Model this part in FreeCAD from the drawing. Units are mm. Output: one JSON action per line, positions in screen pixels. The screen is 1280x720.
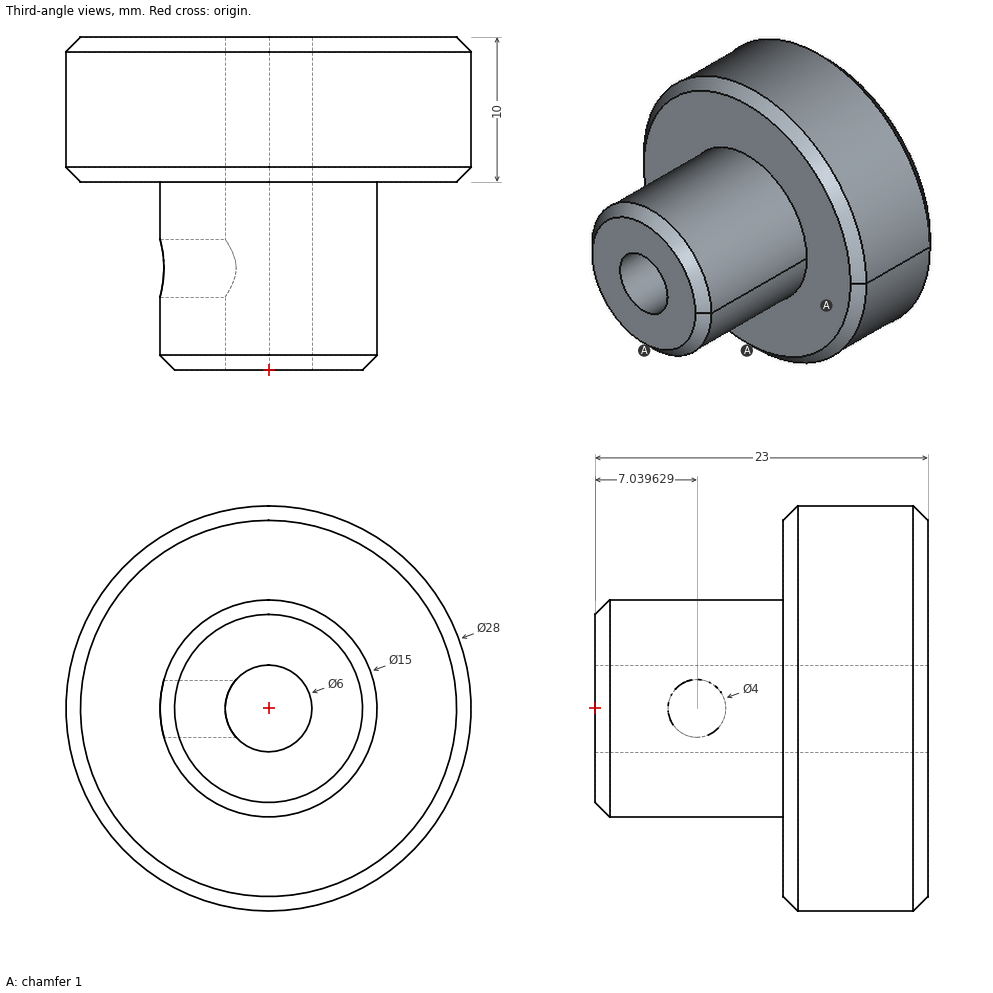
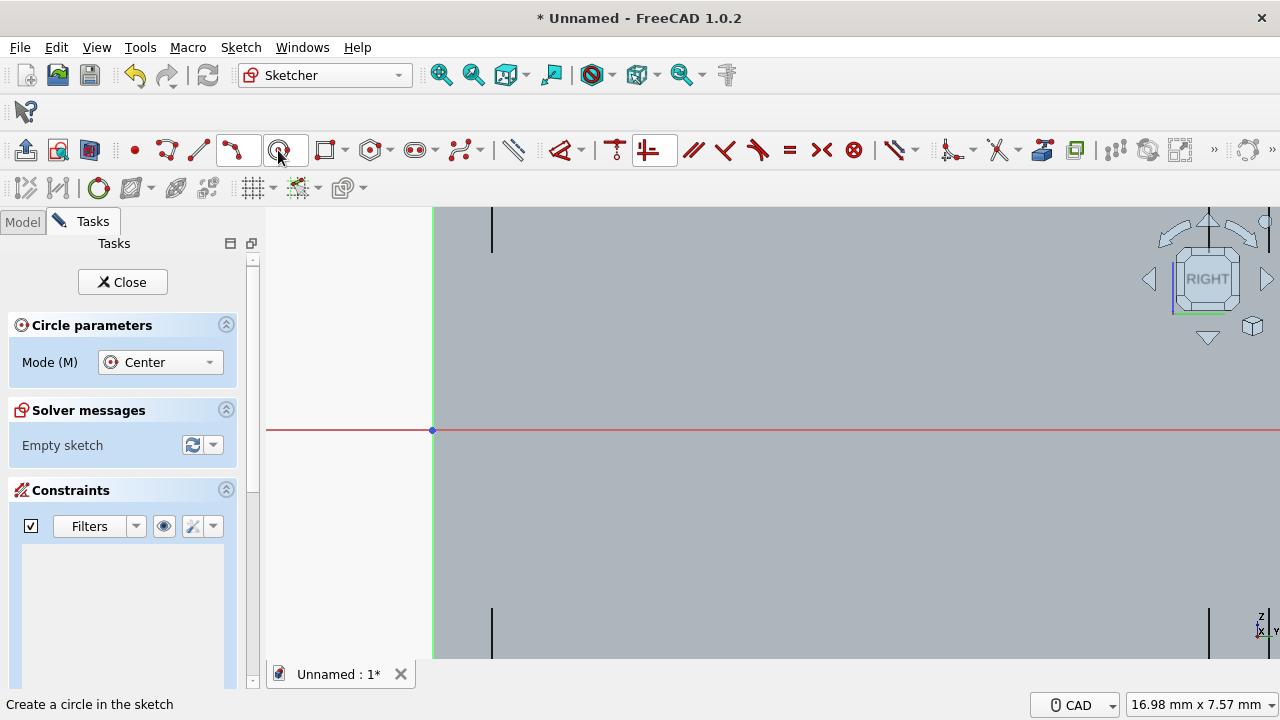
{"action": "left_click", "coordinate": [853, 430]}
{"action": "mouse_move", "coordinate": [937, 346]}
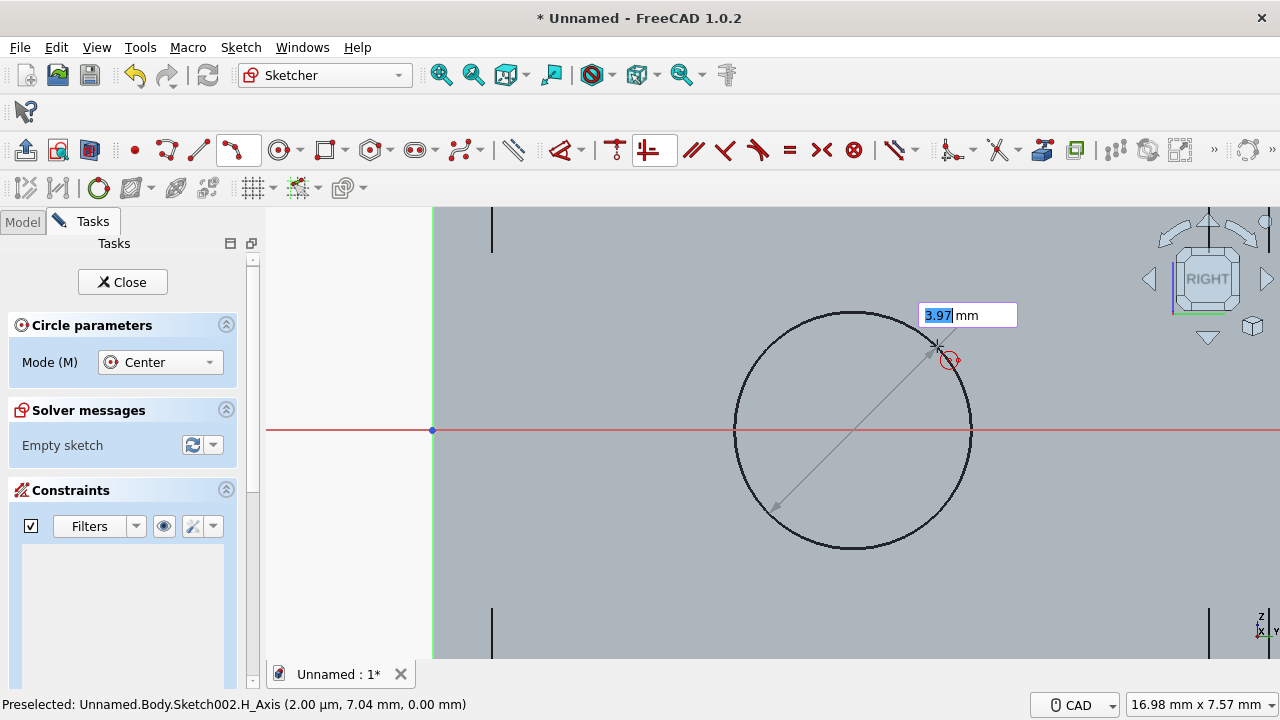
{"action": "type", "text": "4"}
{"action": "key", "text": "Return"}
{"action": "key", "text": "Escape"}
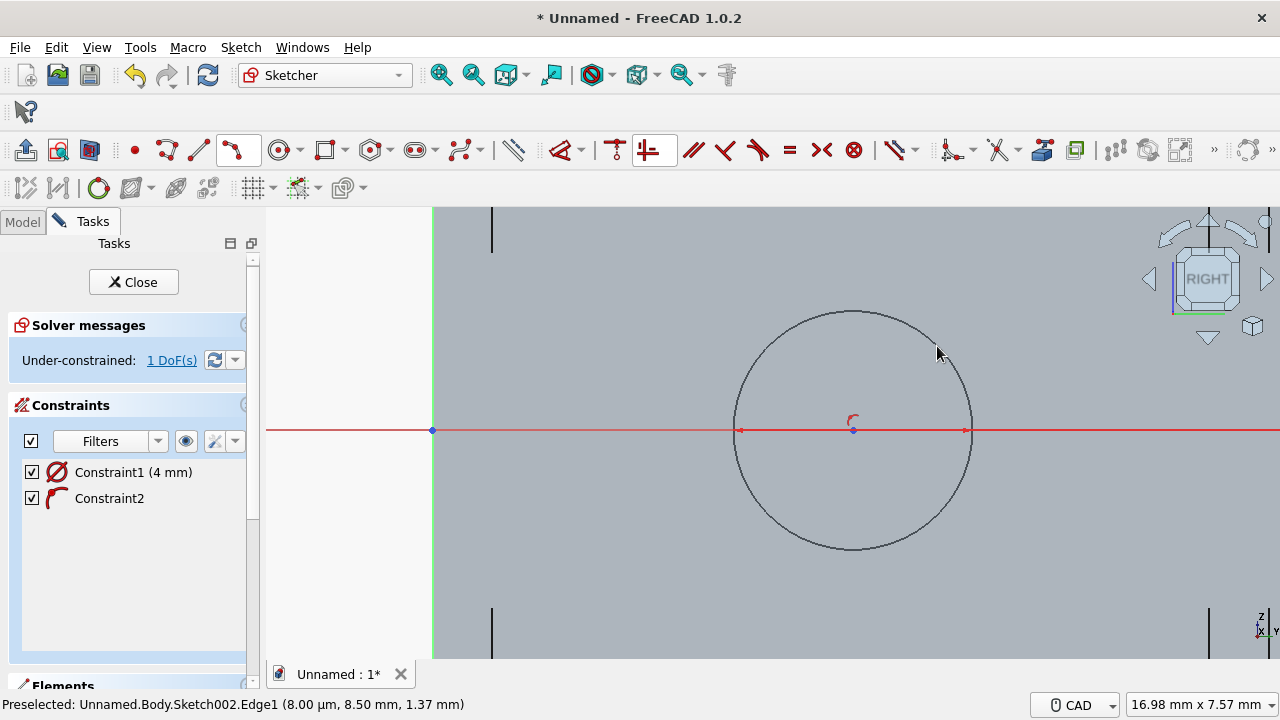
{"action": "key", "text": "d"}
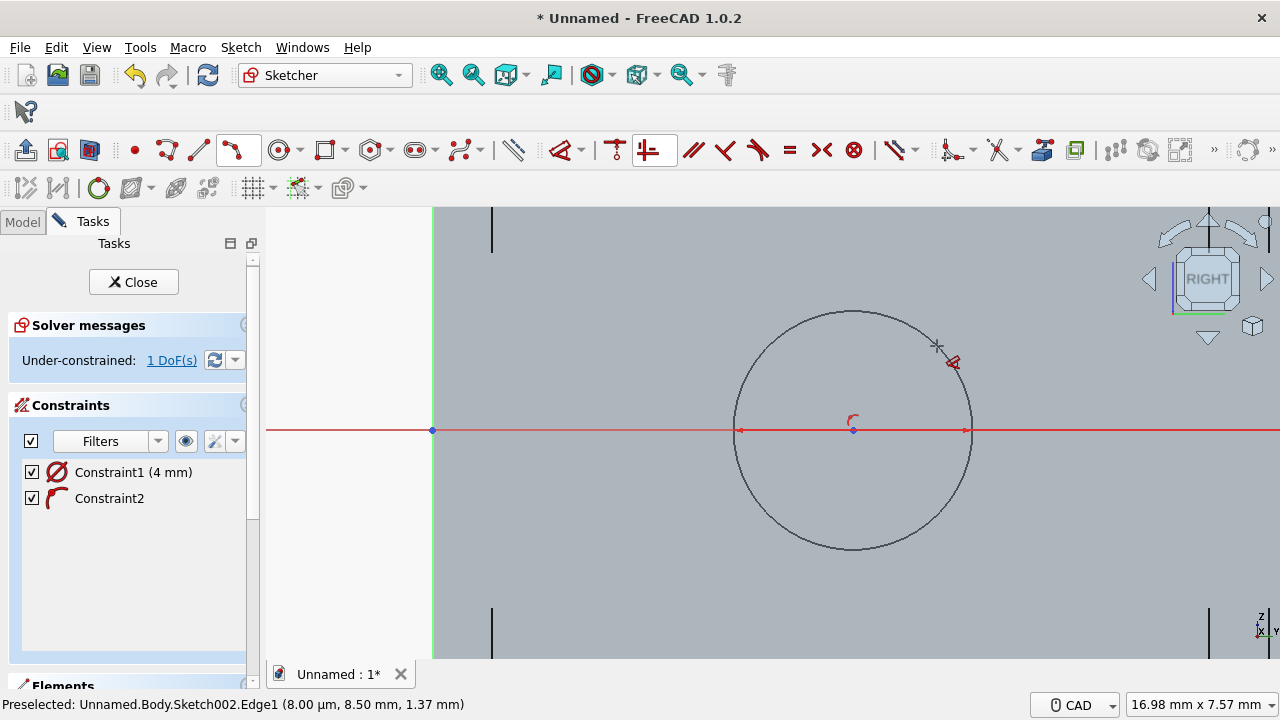
{"action": "left_click", "coordinate": [853, 430]}
{"action": "left_click", "coordinate": [643, 464]}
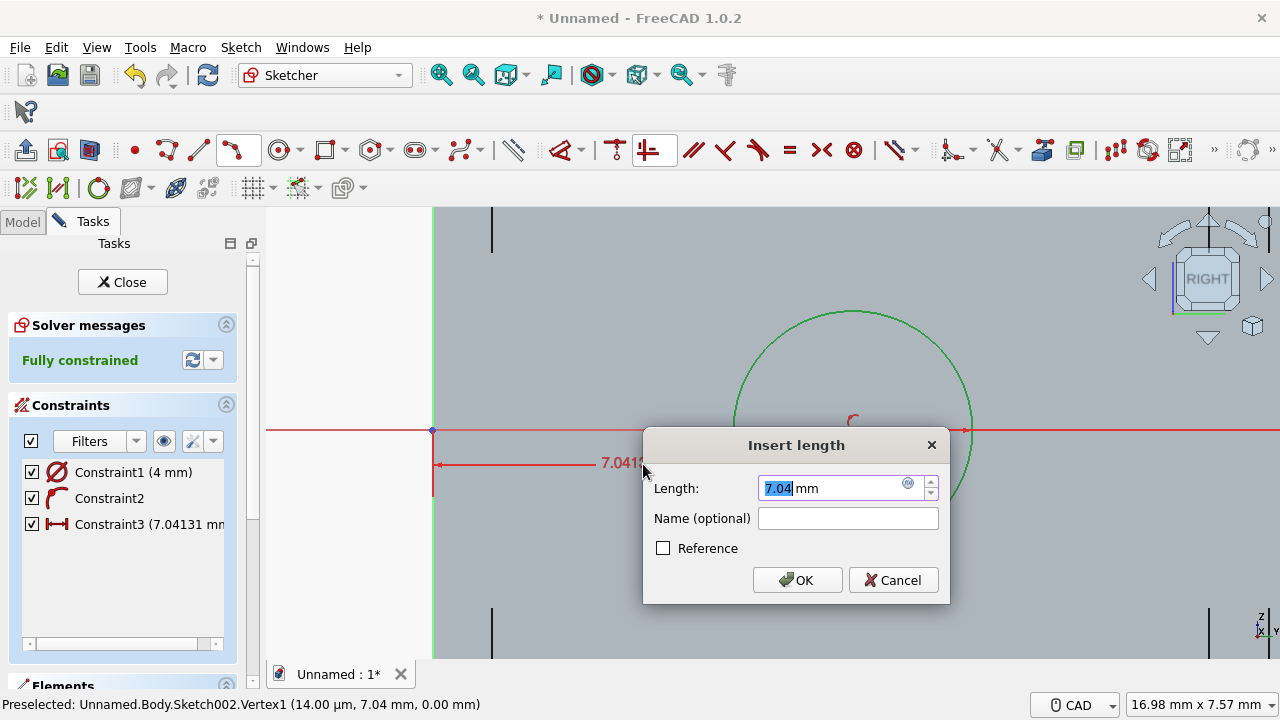
{"action": "type", "text": "7.039629"}
{"action": "key", "text": "Return"}
{"action": "key", "text": "Escape"}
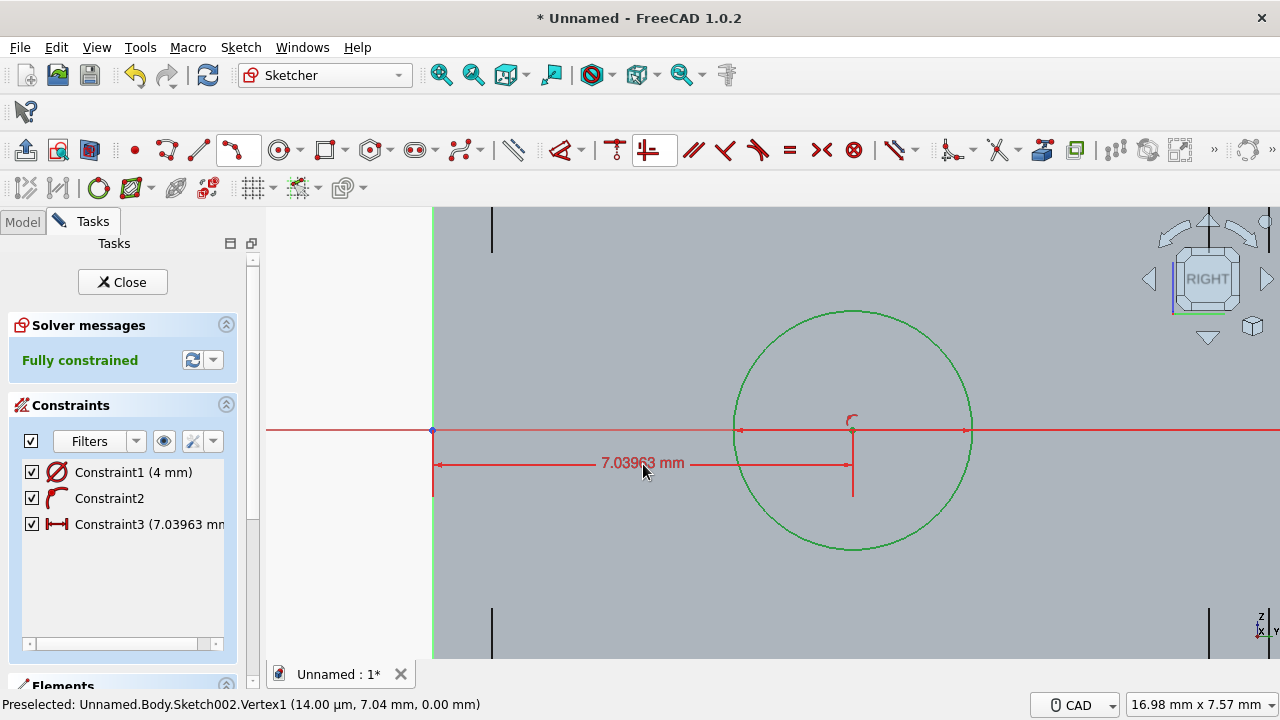
{"action": "left_click", "coordinate": [123, 282]}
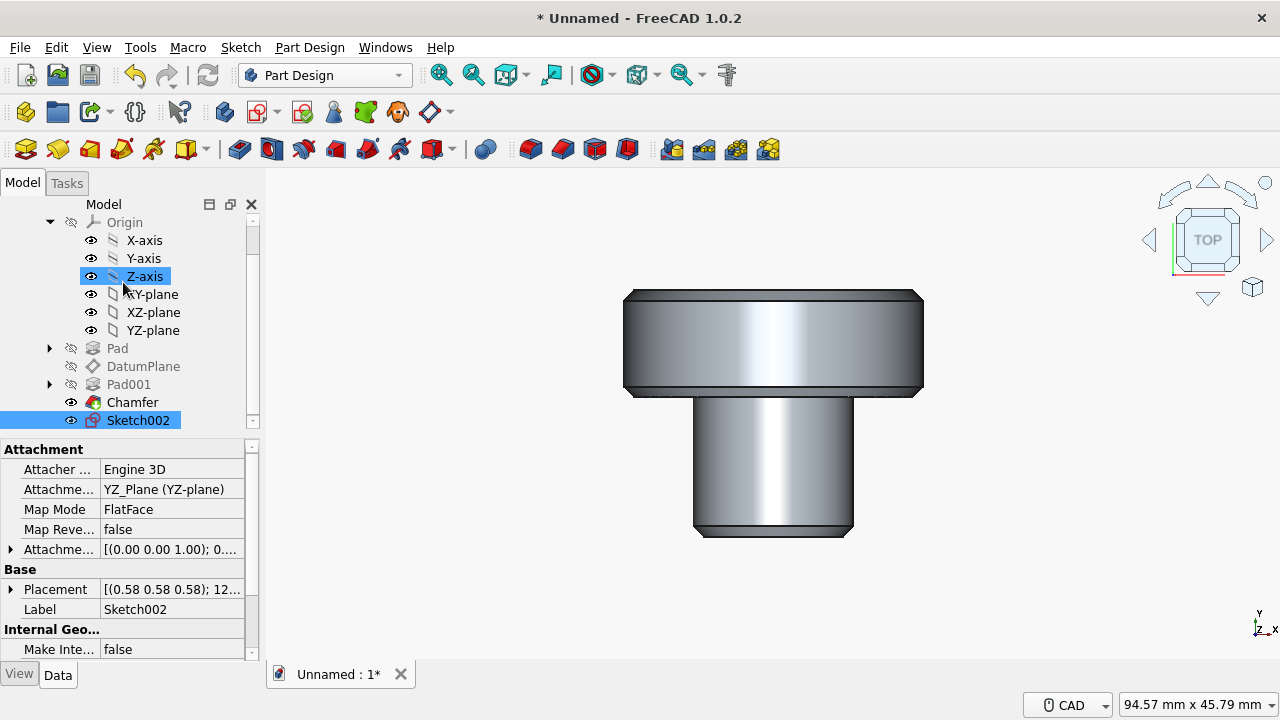
{"action": "left_click", "coordinate": [240, 150]}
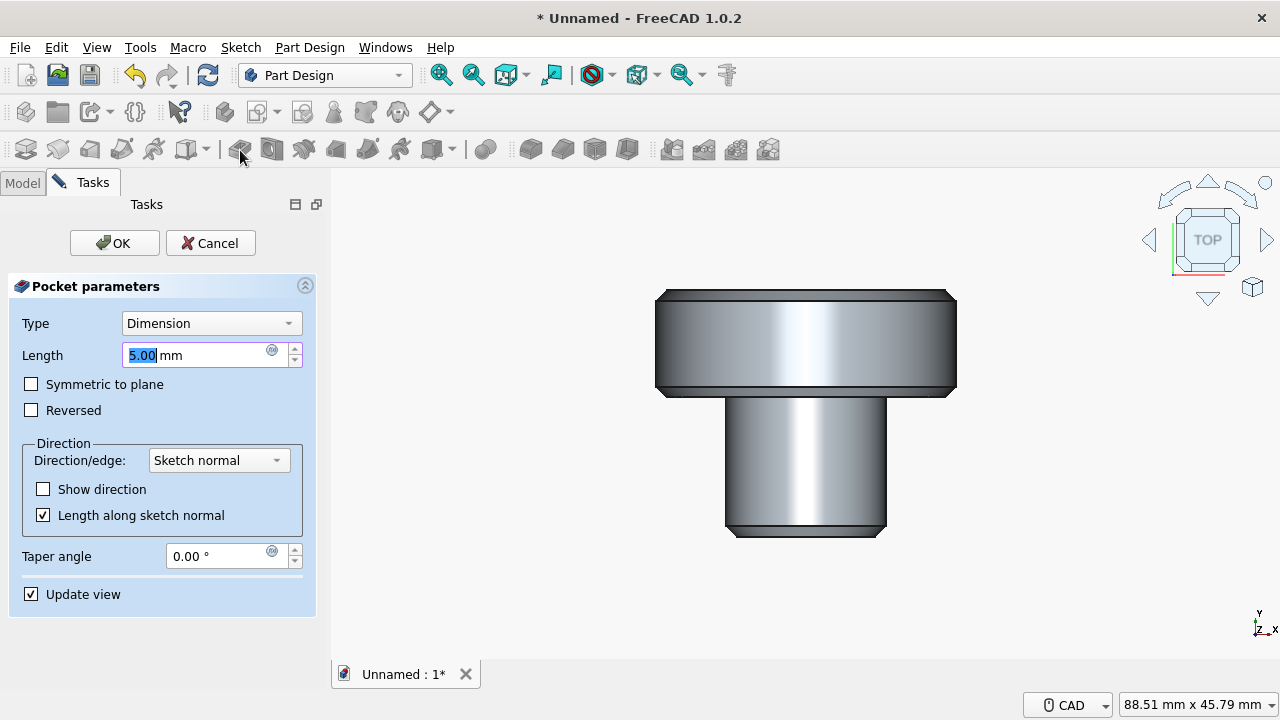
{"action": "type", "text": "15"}
{"action": "key", "text": "Tab"}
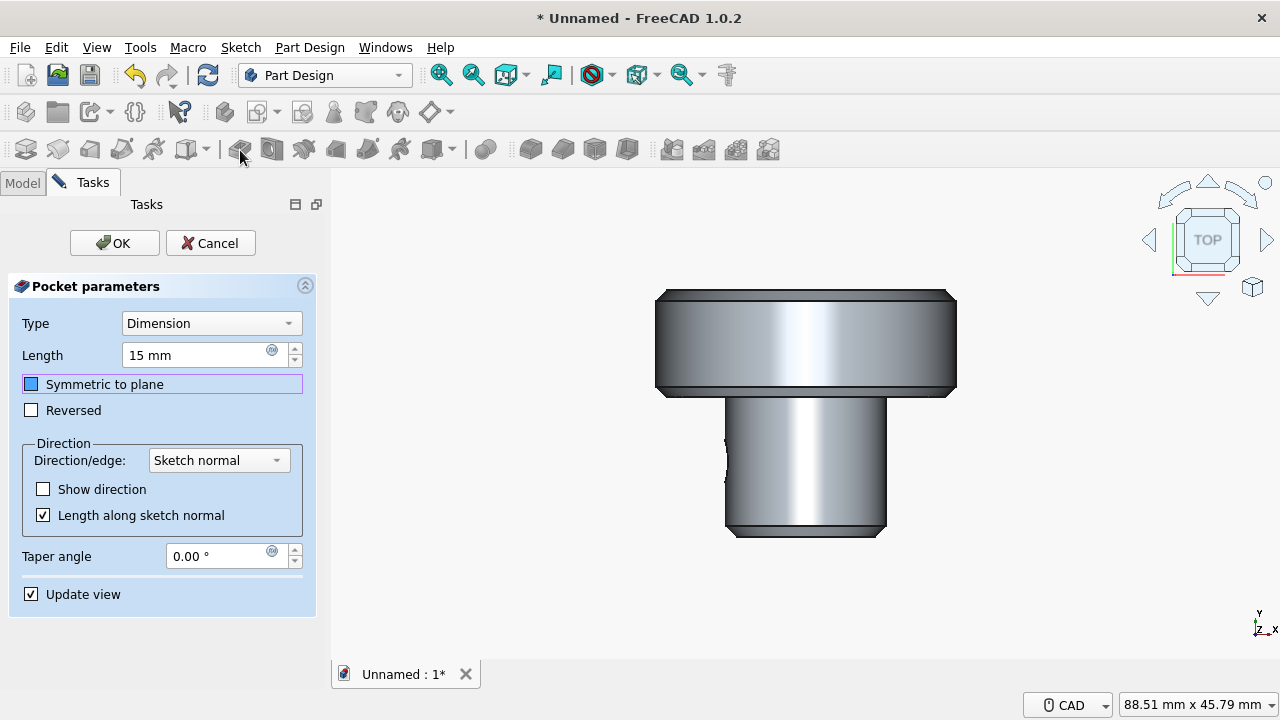
{"action": "left_click", "coordinate": [115, 243]}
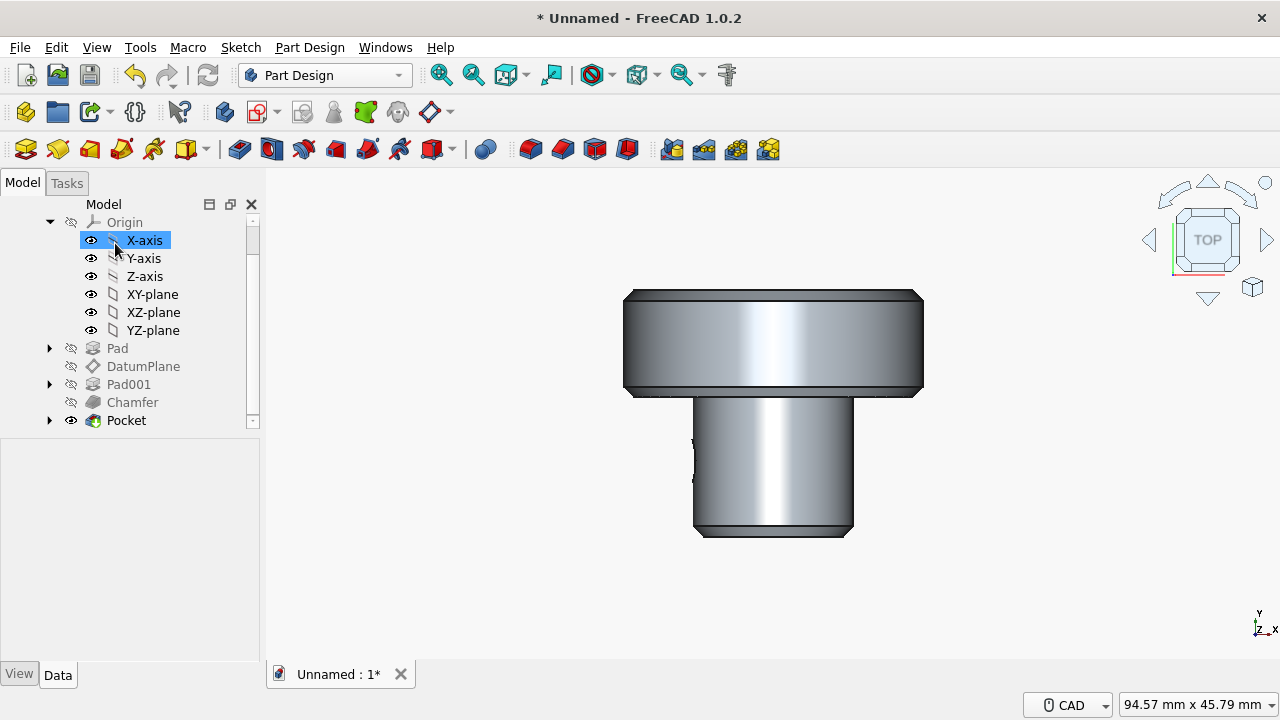
{"action": "key", "text": "0"}